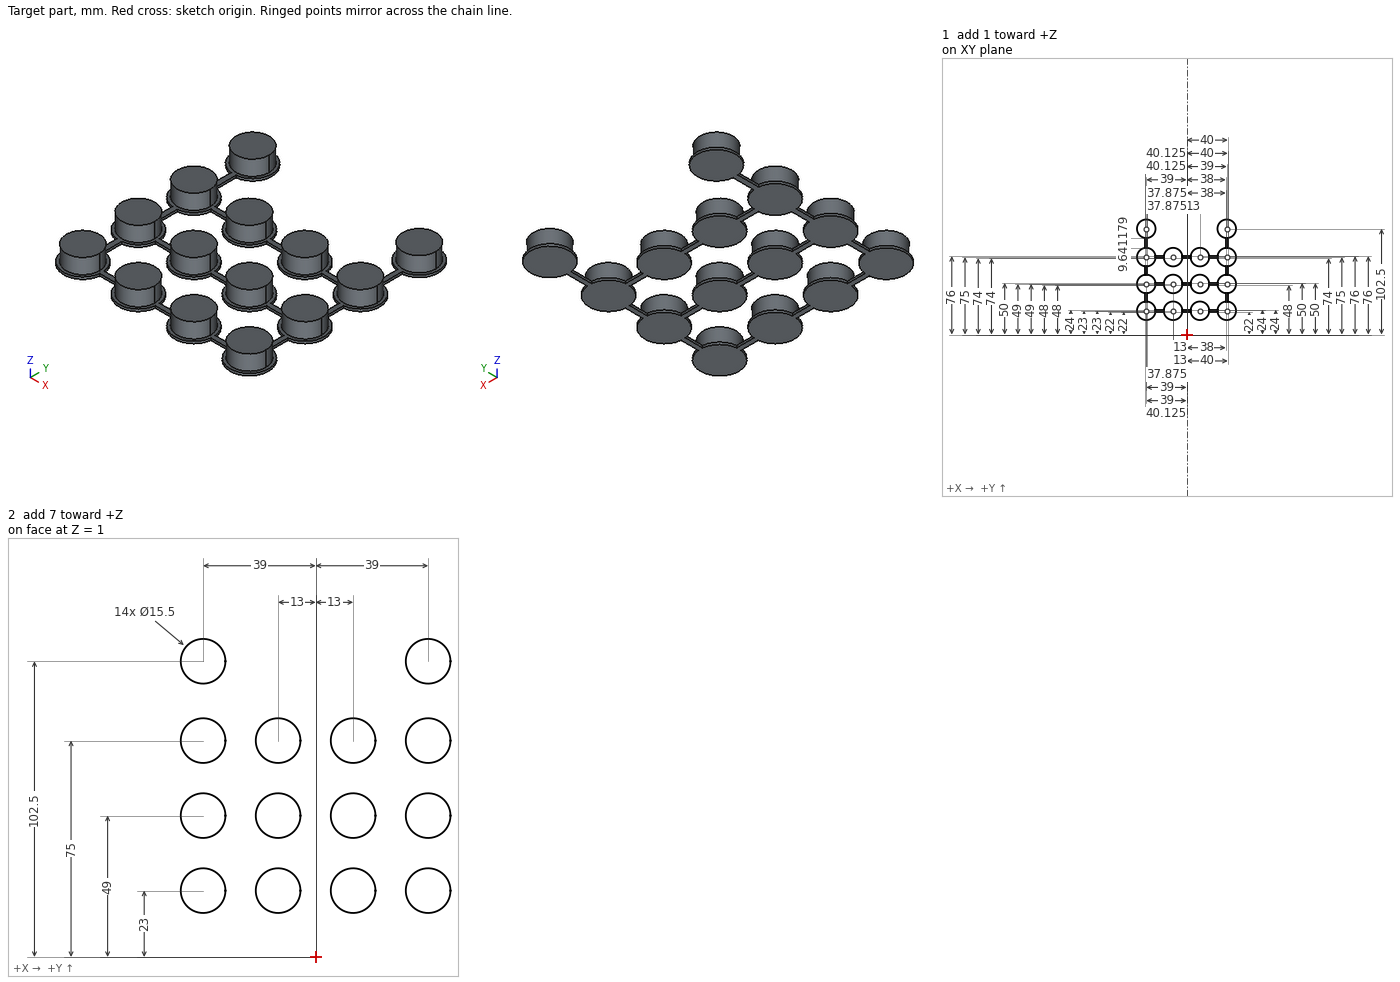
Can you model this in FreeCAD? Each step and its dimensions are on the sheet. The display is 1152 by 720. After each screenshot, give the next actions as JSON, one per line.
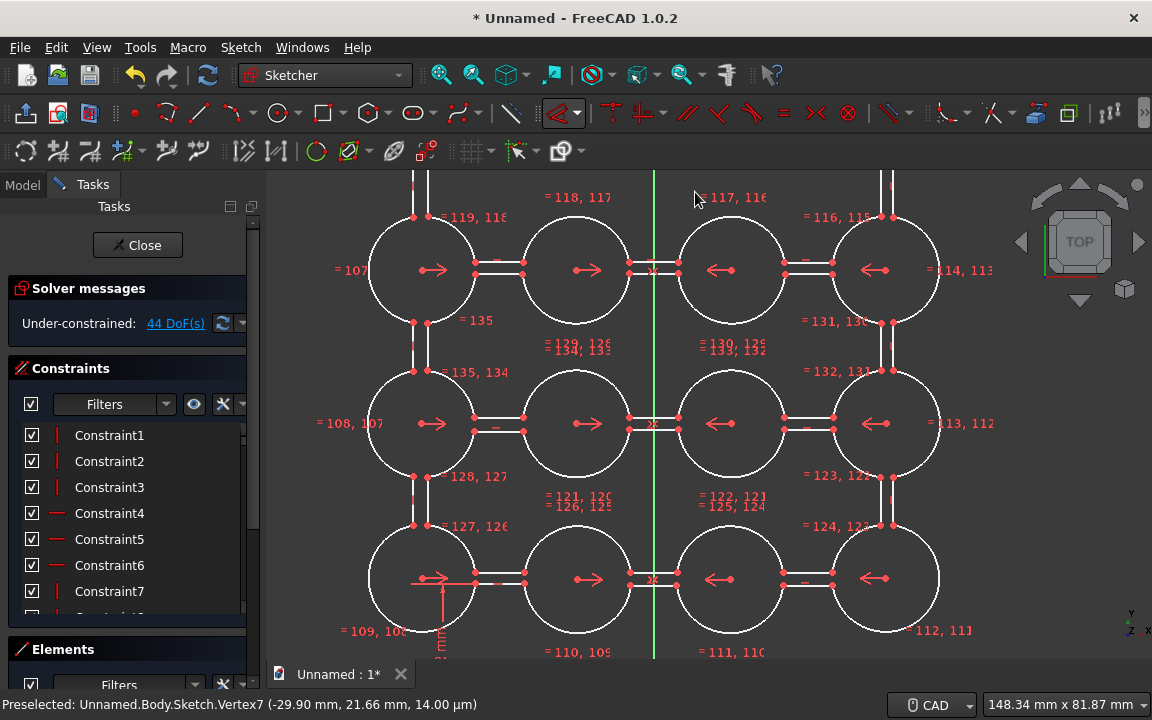
{"action": "left_click", "coordinate": [631, 586]}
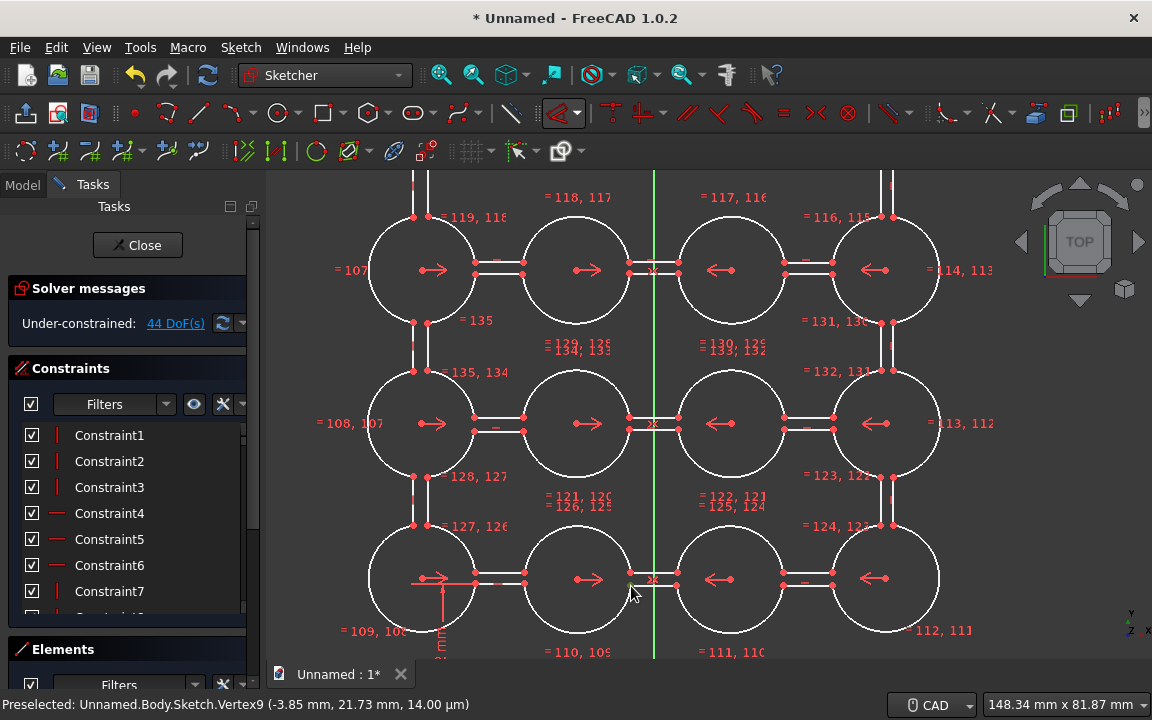
{"action": "left_click", "coordinate": [580, 114]}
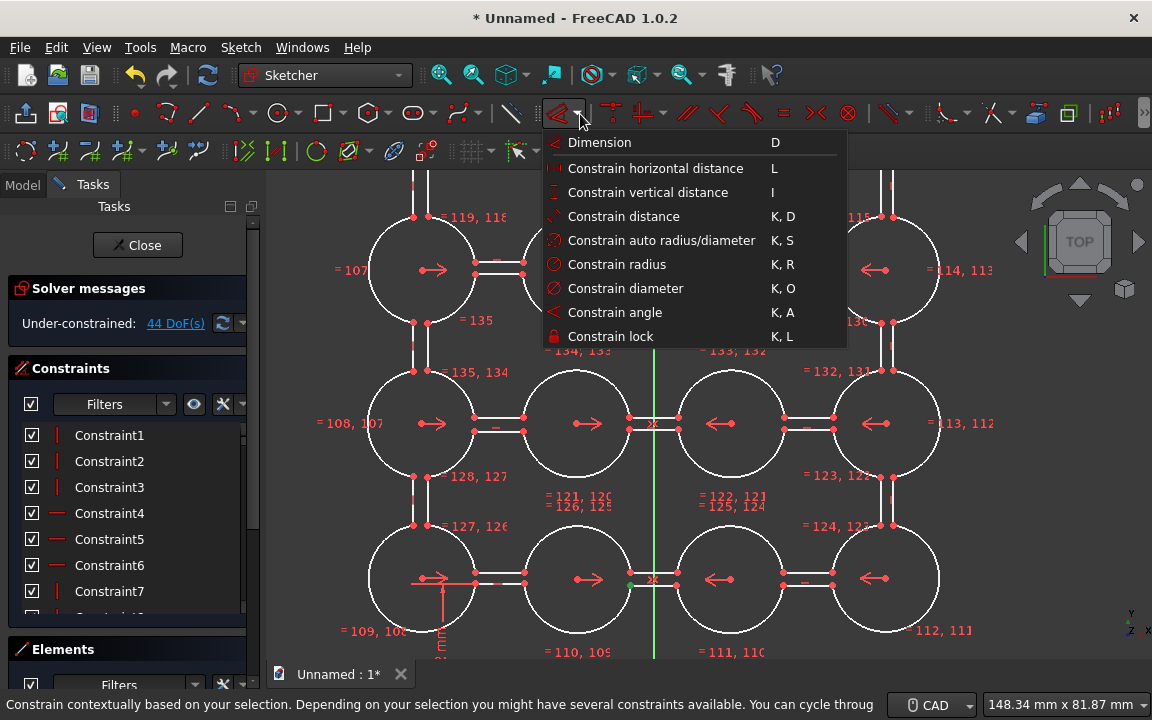
{"action": "left_click", "coordinate": [695, 192]}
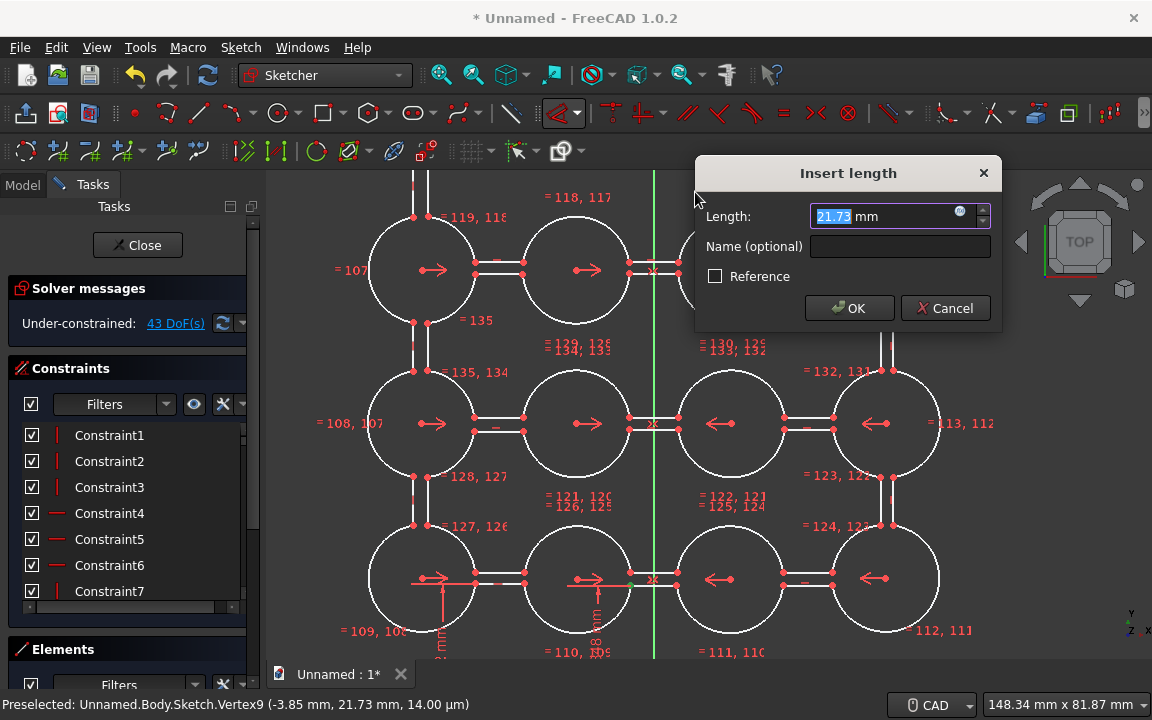
{"action": "type", "text": "22"}
{"action": "key", "text": "Return"}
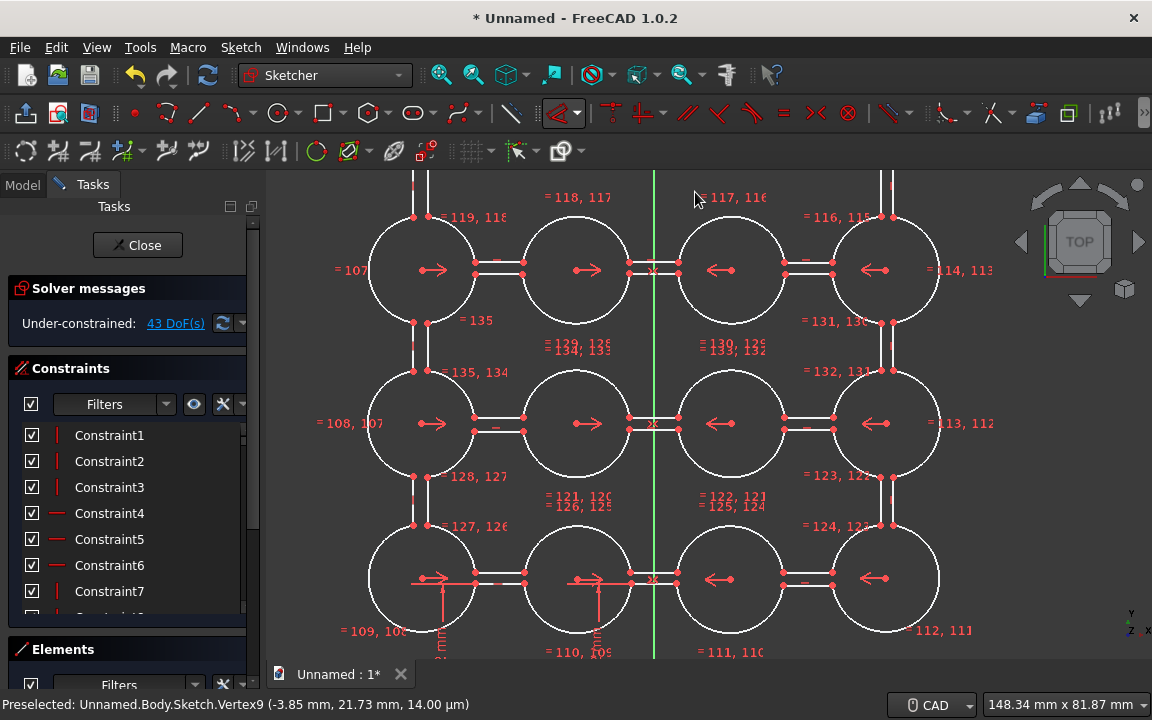
{"action": "left_click", "coordinate": [783, 586]}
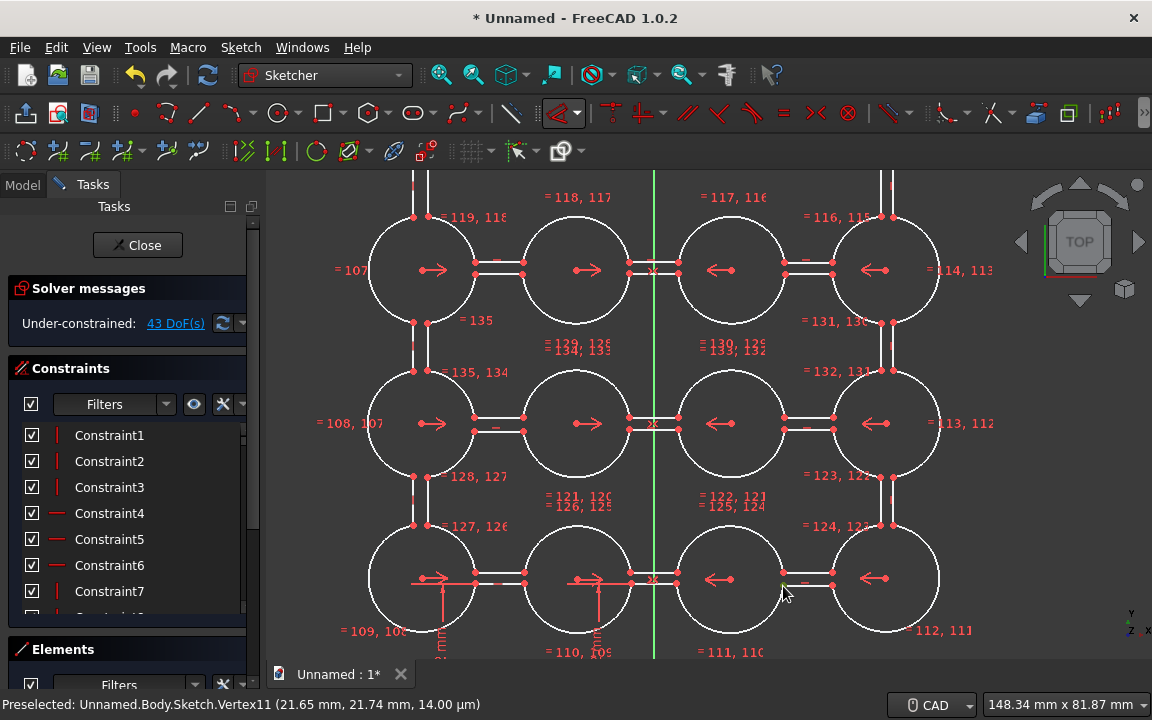
{"action": "key", "text": "i"}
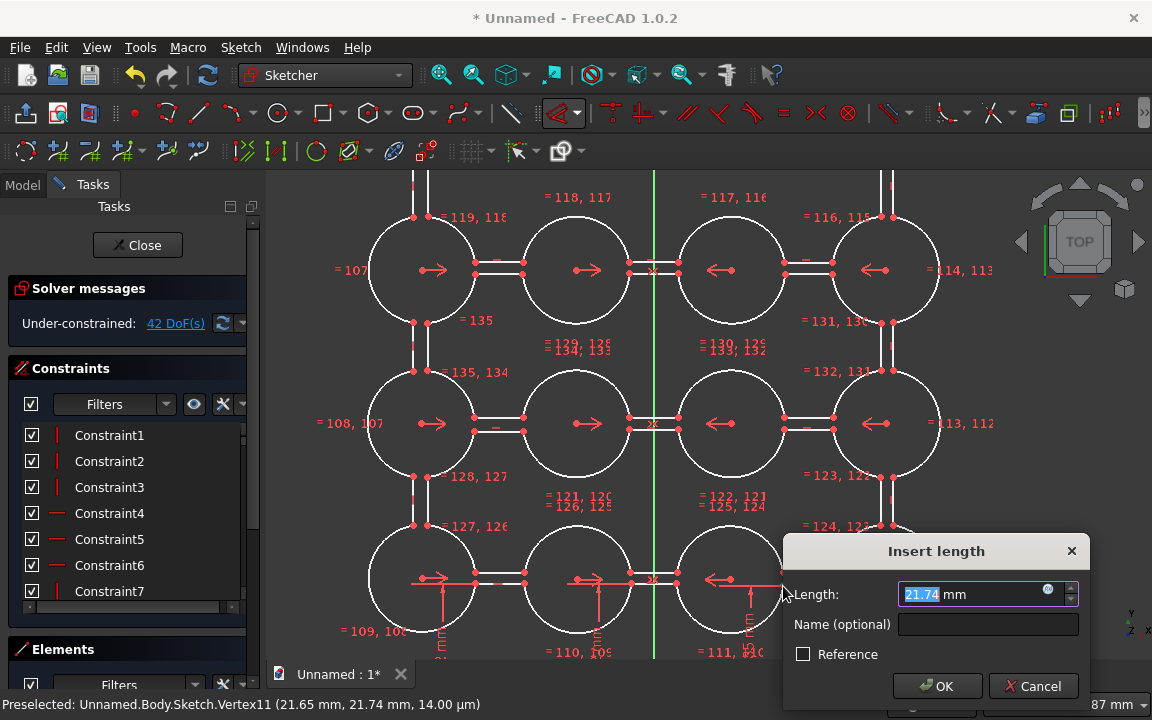
{"action": "type", "text": "22"}
{"action": "key", "text": "Return"}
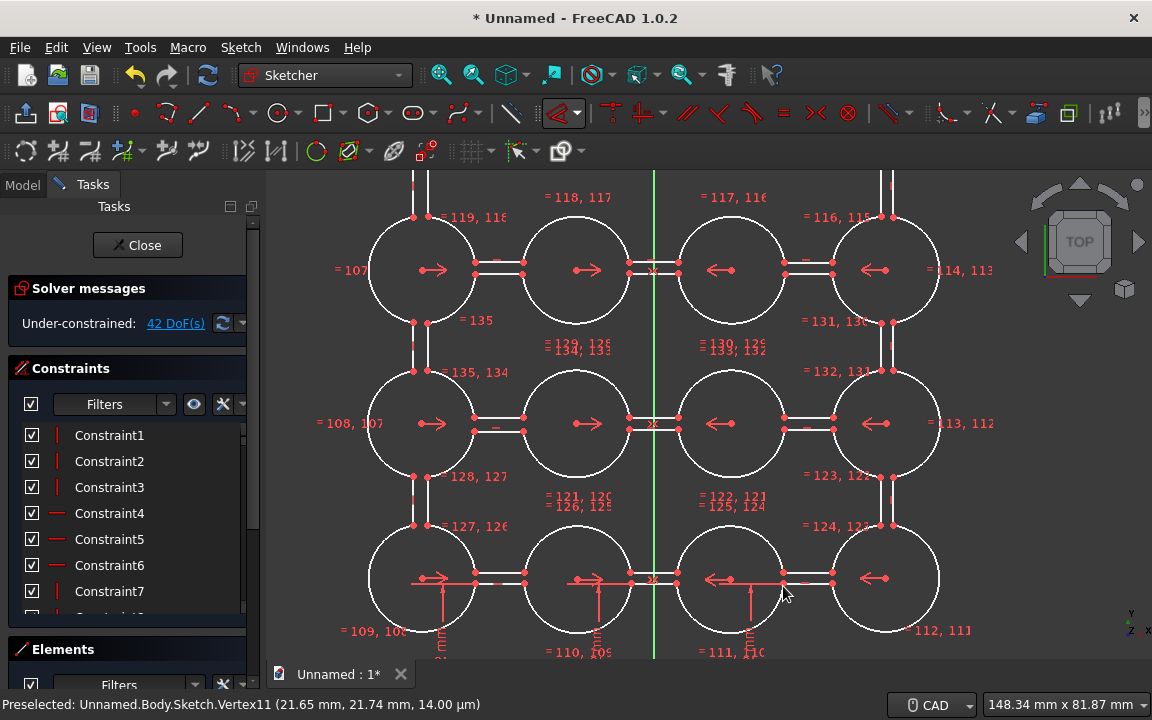
{"action": "left_click", "coordinate": [893, 525]}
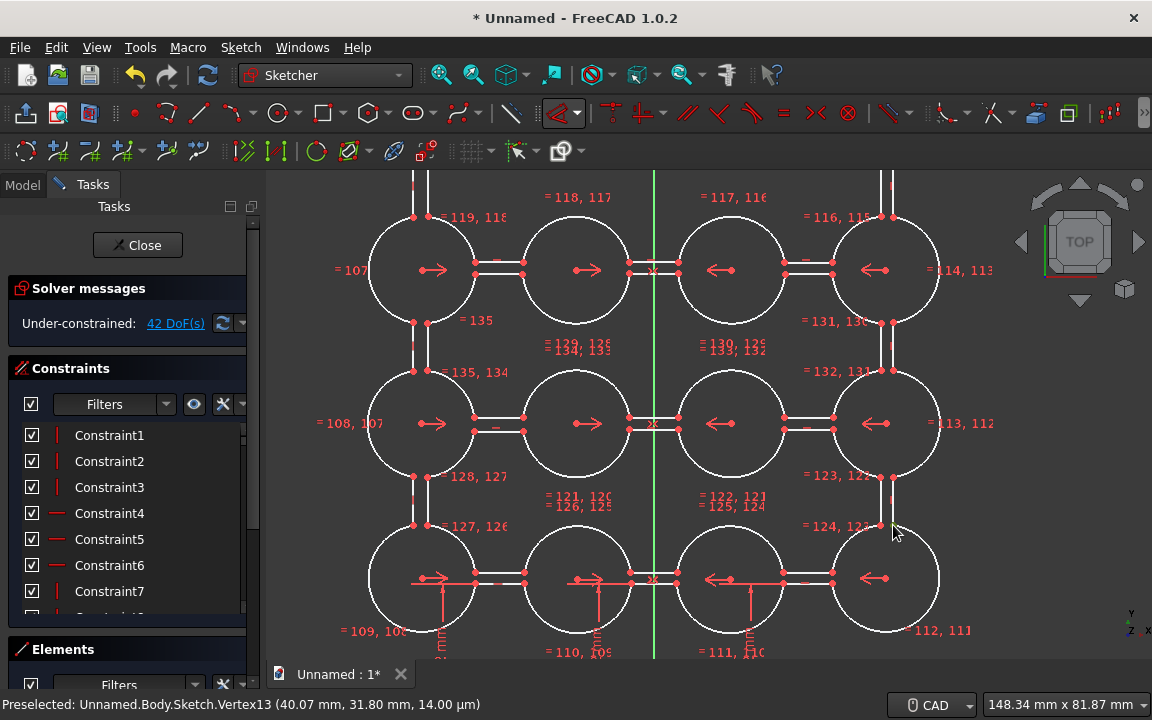
{"action": "left_click", "coordinate": [580, 114]}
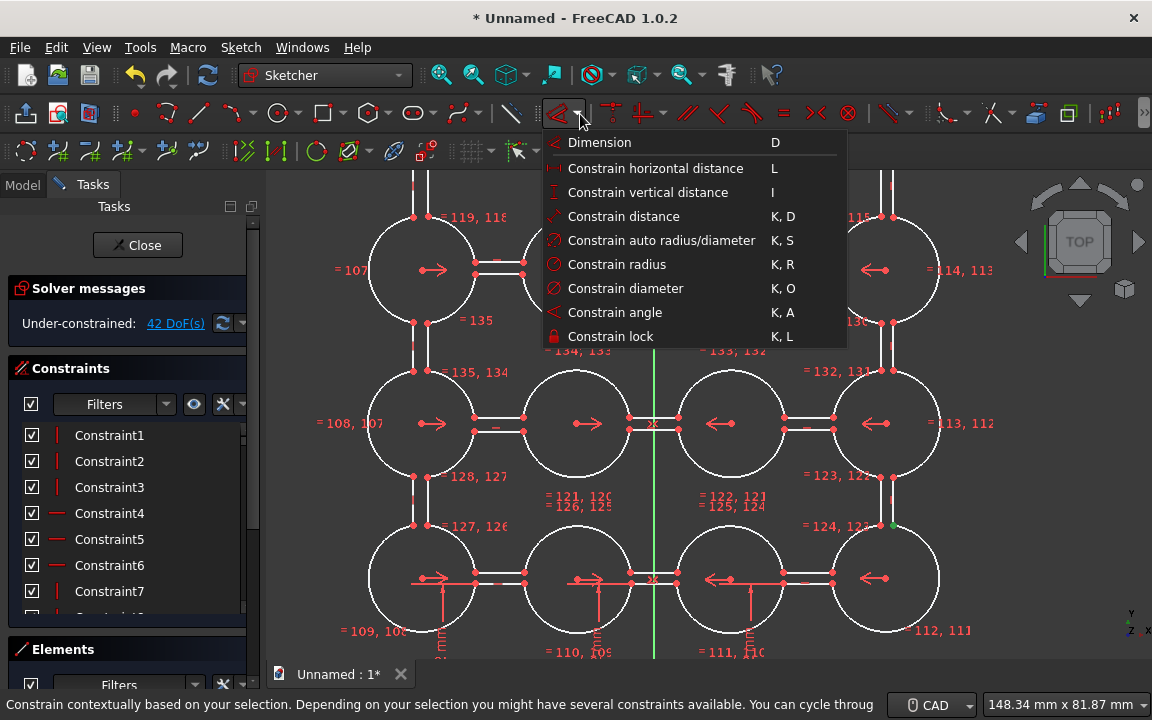
{"action": "left_click", "coordinate": [695, 168]}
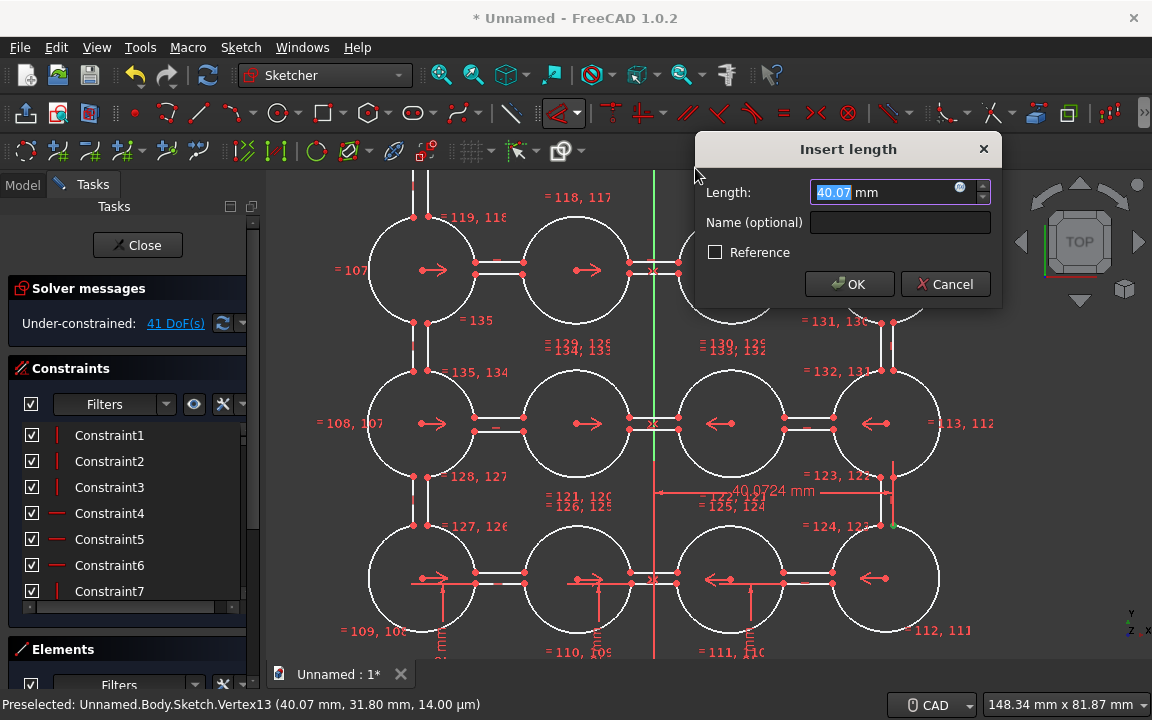
{"action": "type", "text": "40"}
{"action": "key", "text": "Return"}